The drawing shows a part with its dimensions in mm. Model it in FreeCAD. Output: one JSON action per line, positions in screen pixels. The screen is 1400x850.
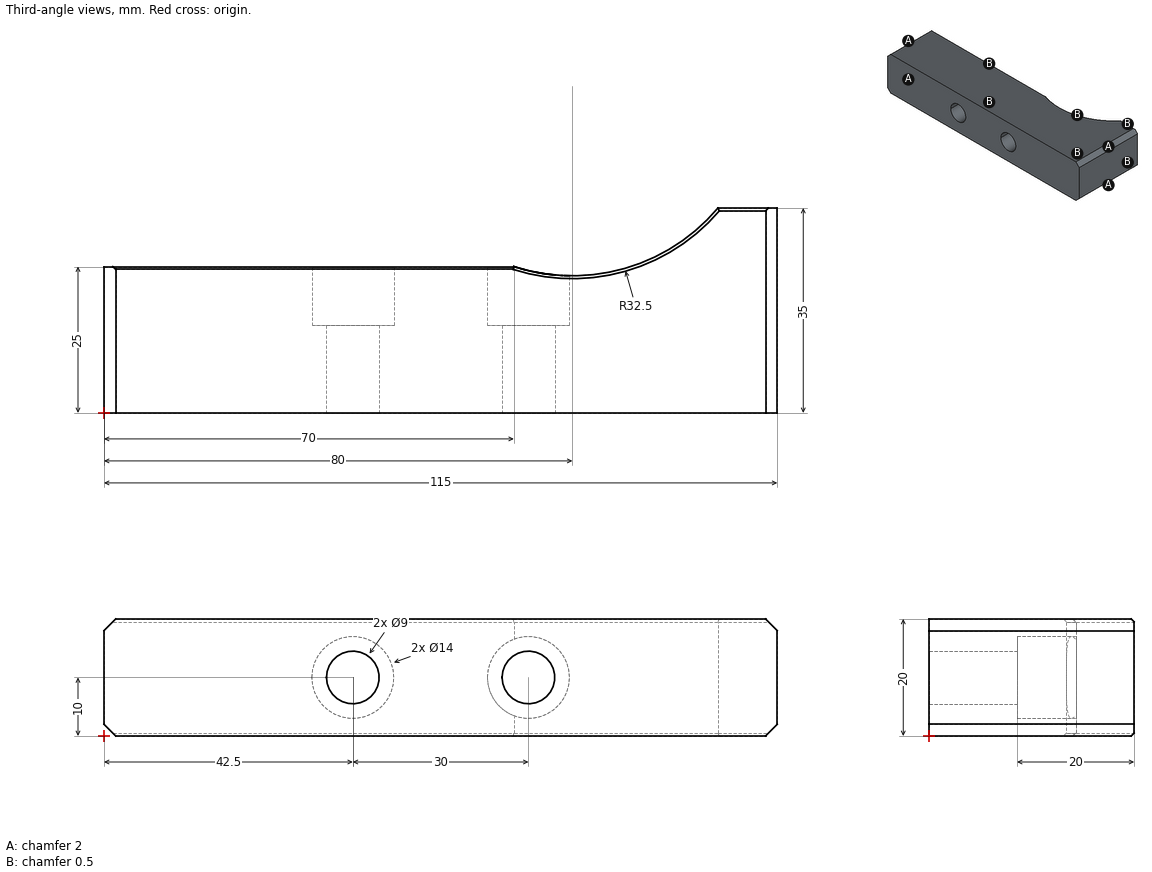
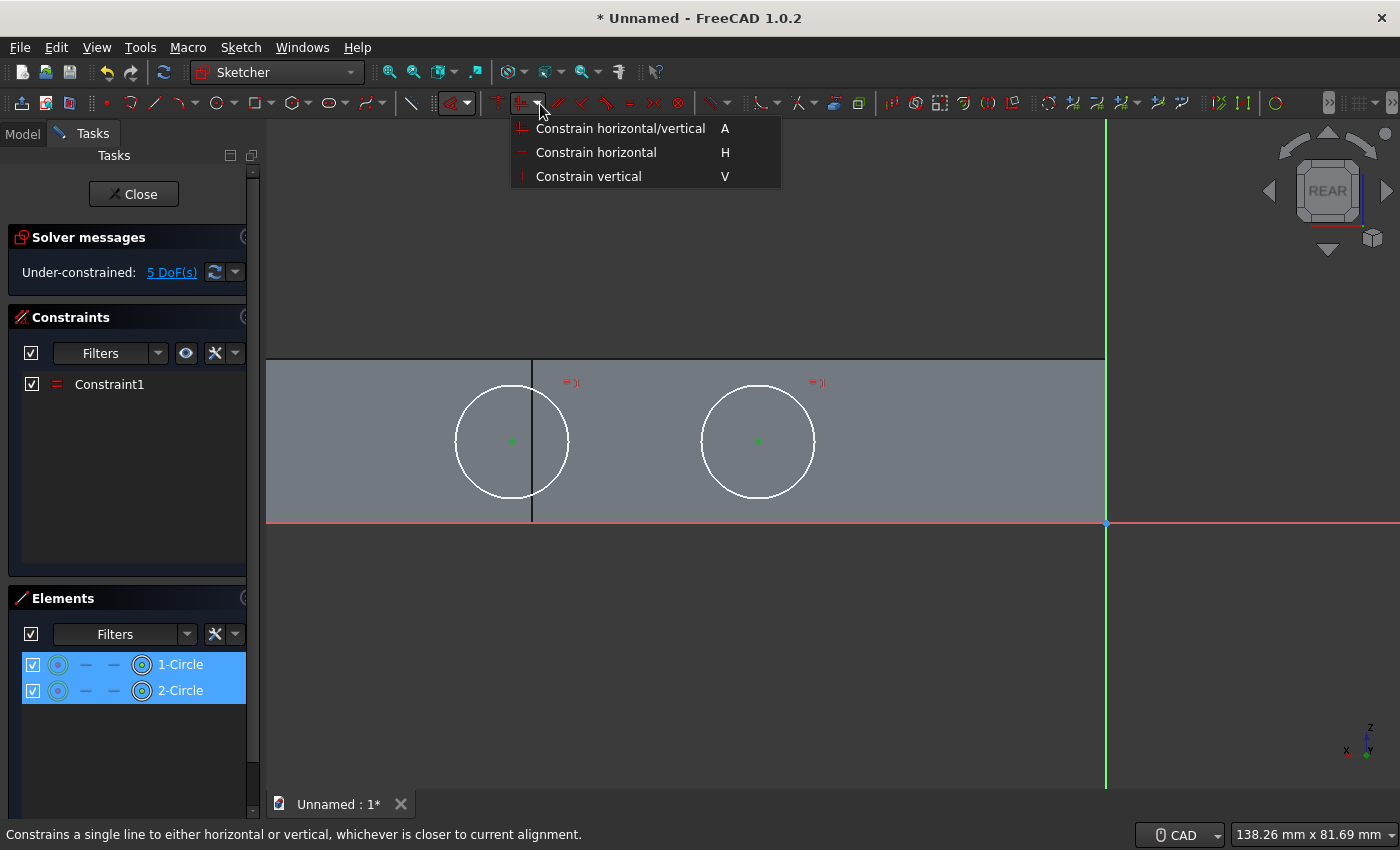
{"action": "left_click", "coordinate": [646, 152]}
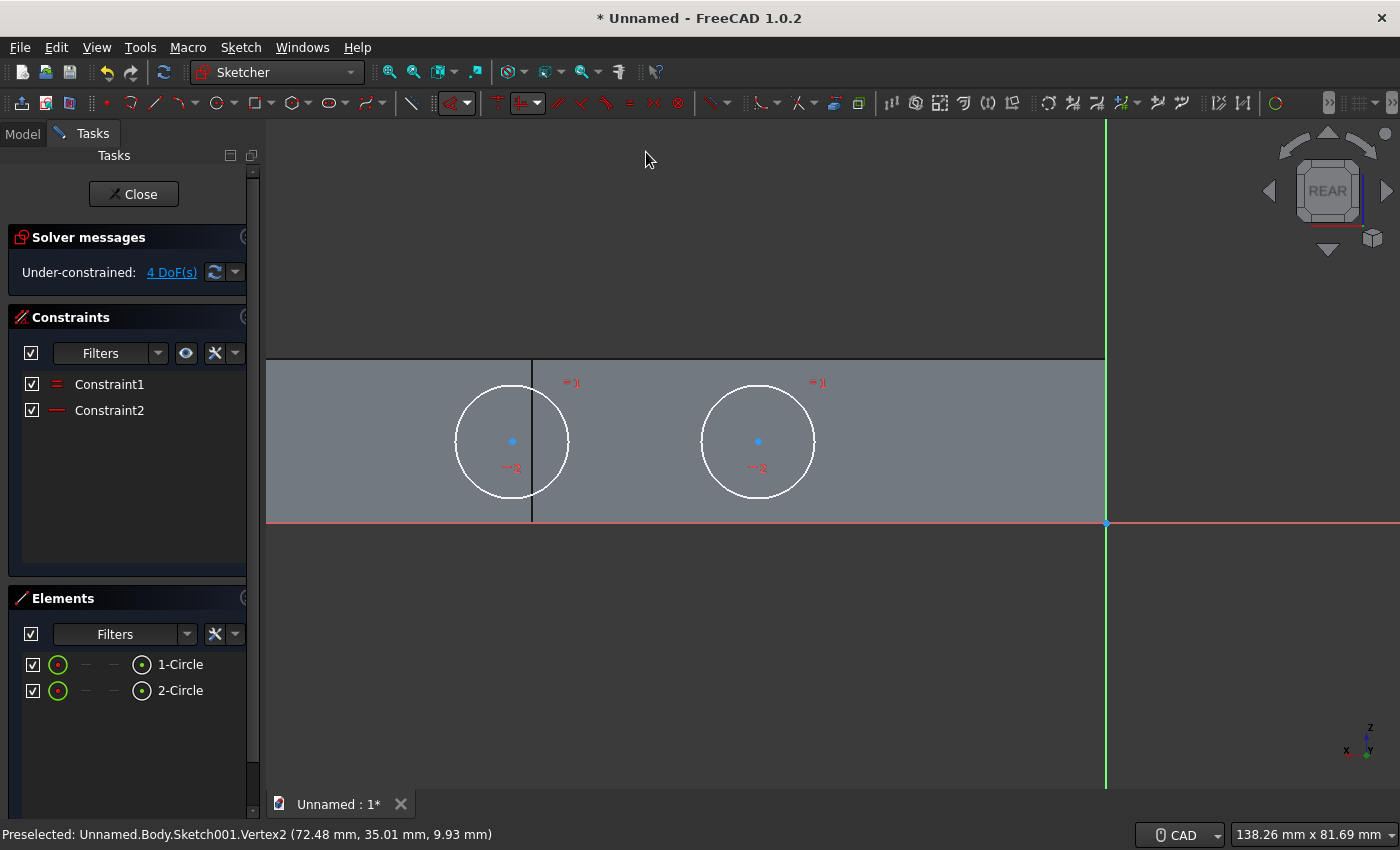
{"action": "left_click", "coordinate": [798, 402]}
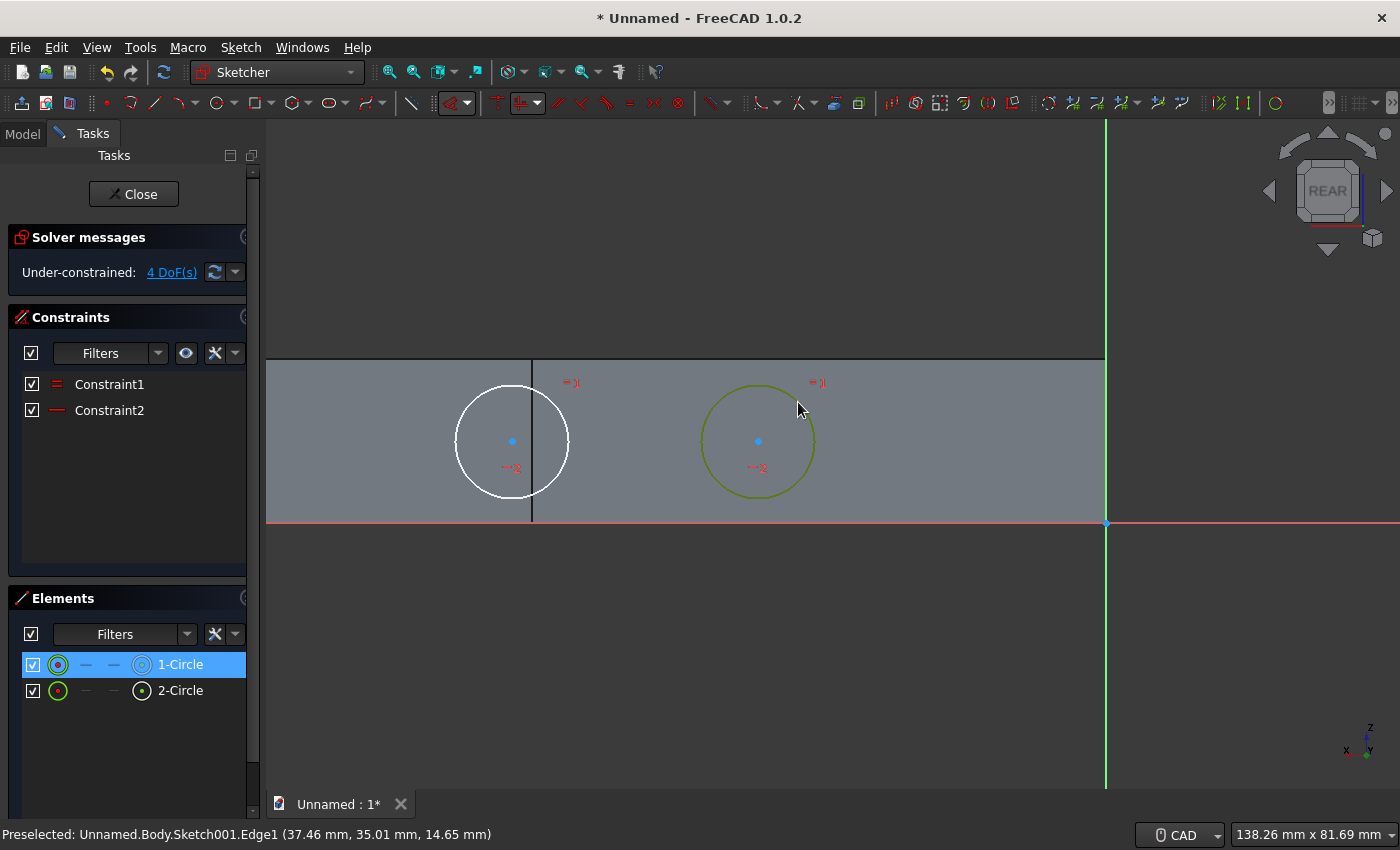
{"action": "left_click", "coordinate": [470, 104]}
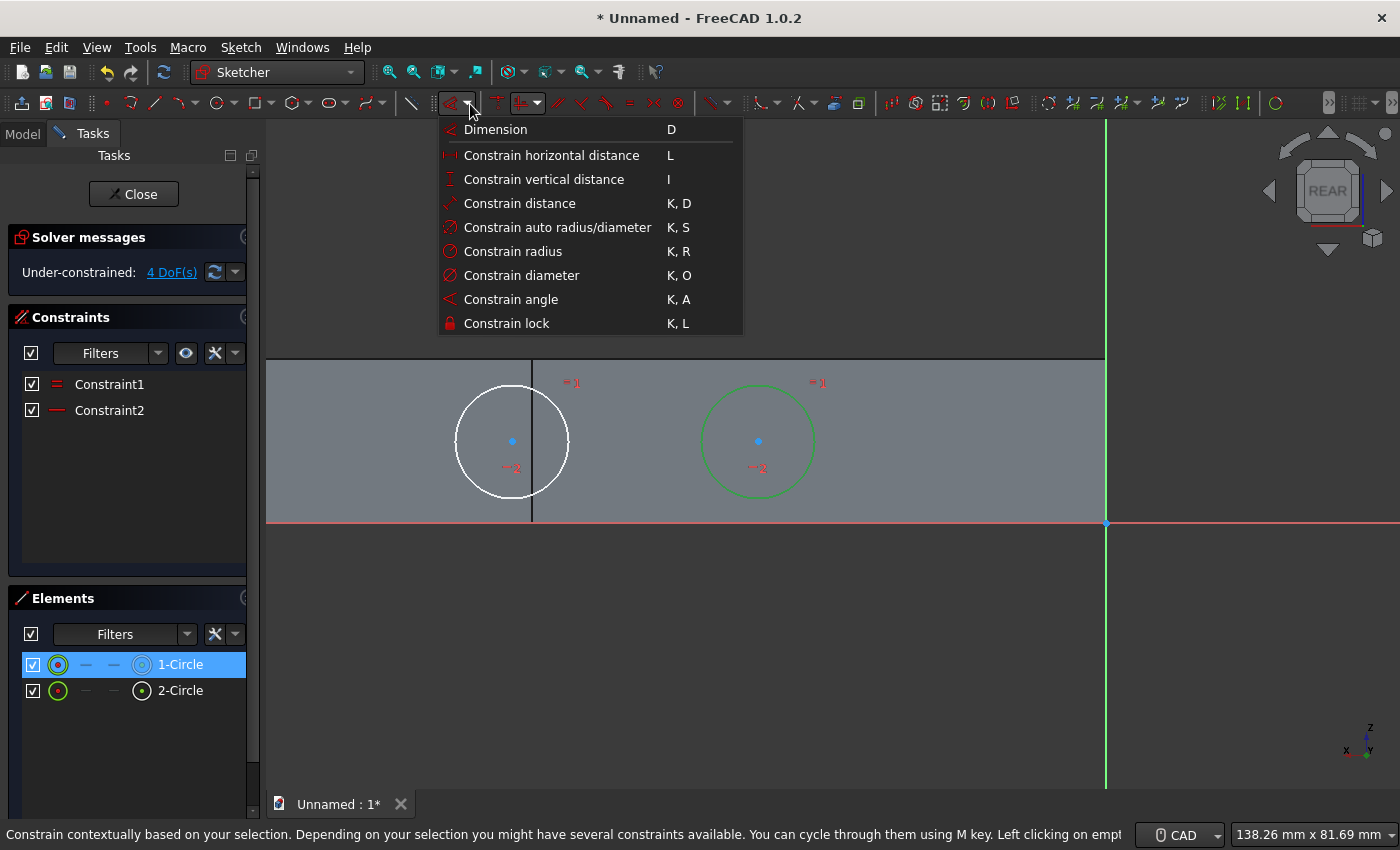
{"action": "left_click", "coordinate": [591, 275]}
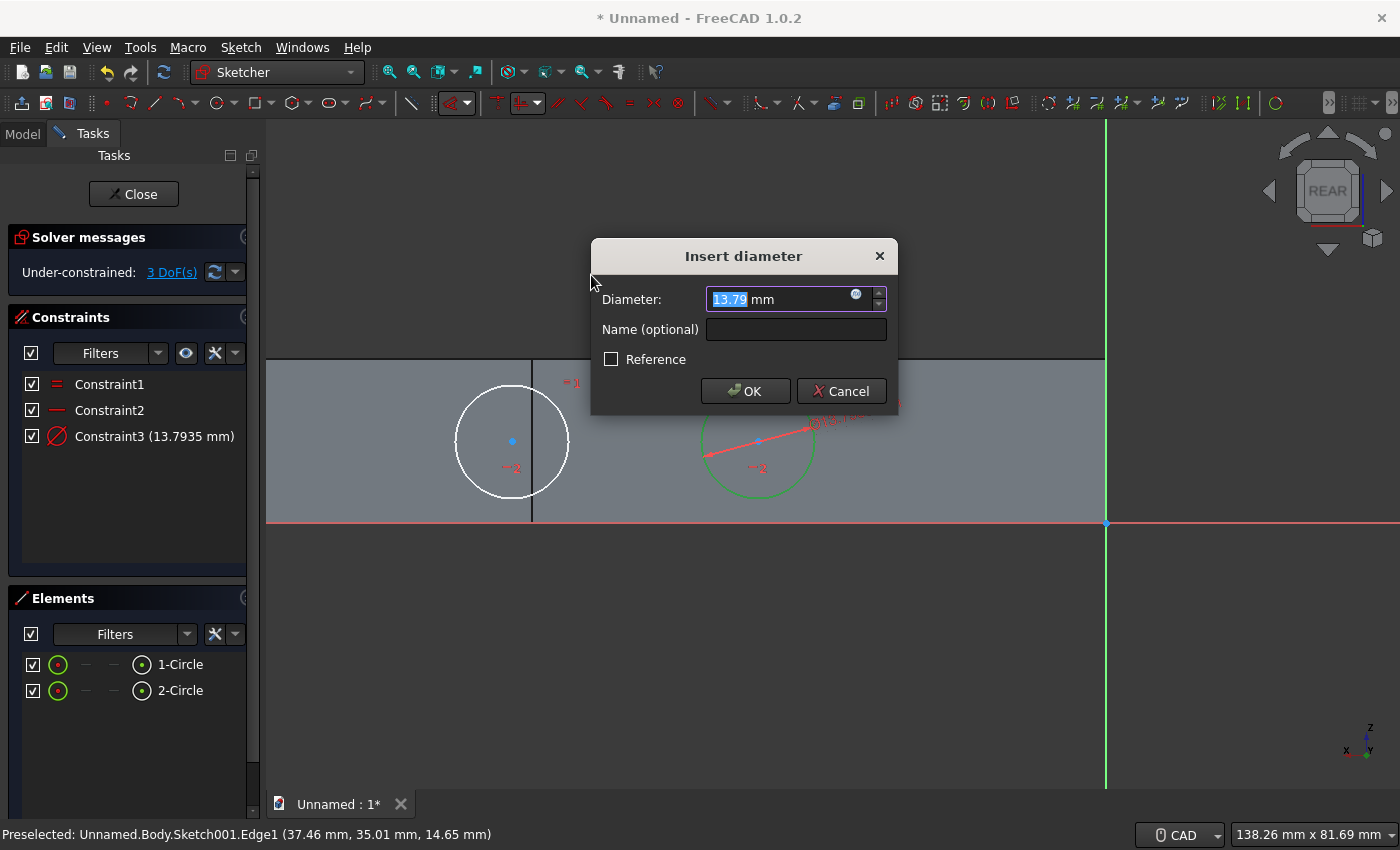
{"action": "type", "text": "14"}
{"action": "key", "text": "Return"}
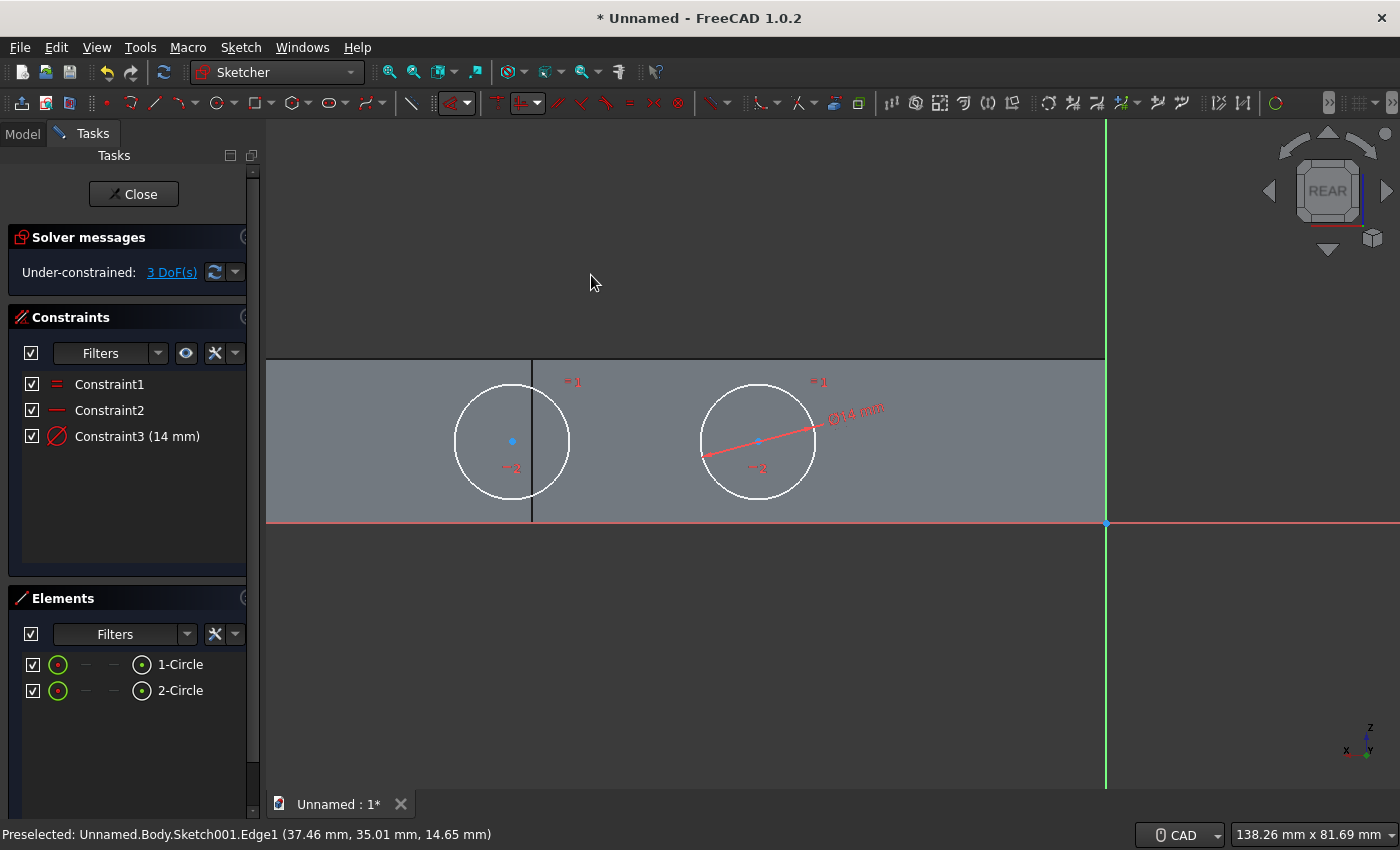
{"action": "left_click", "coordinate": [758, 442]}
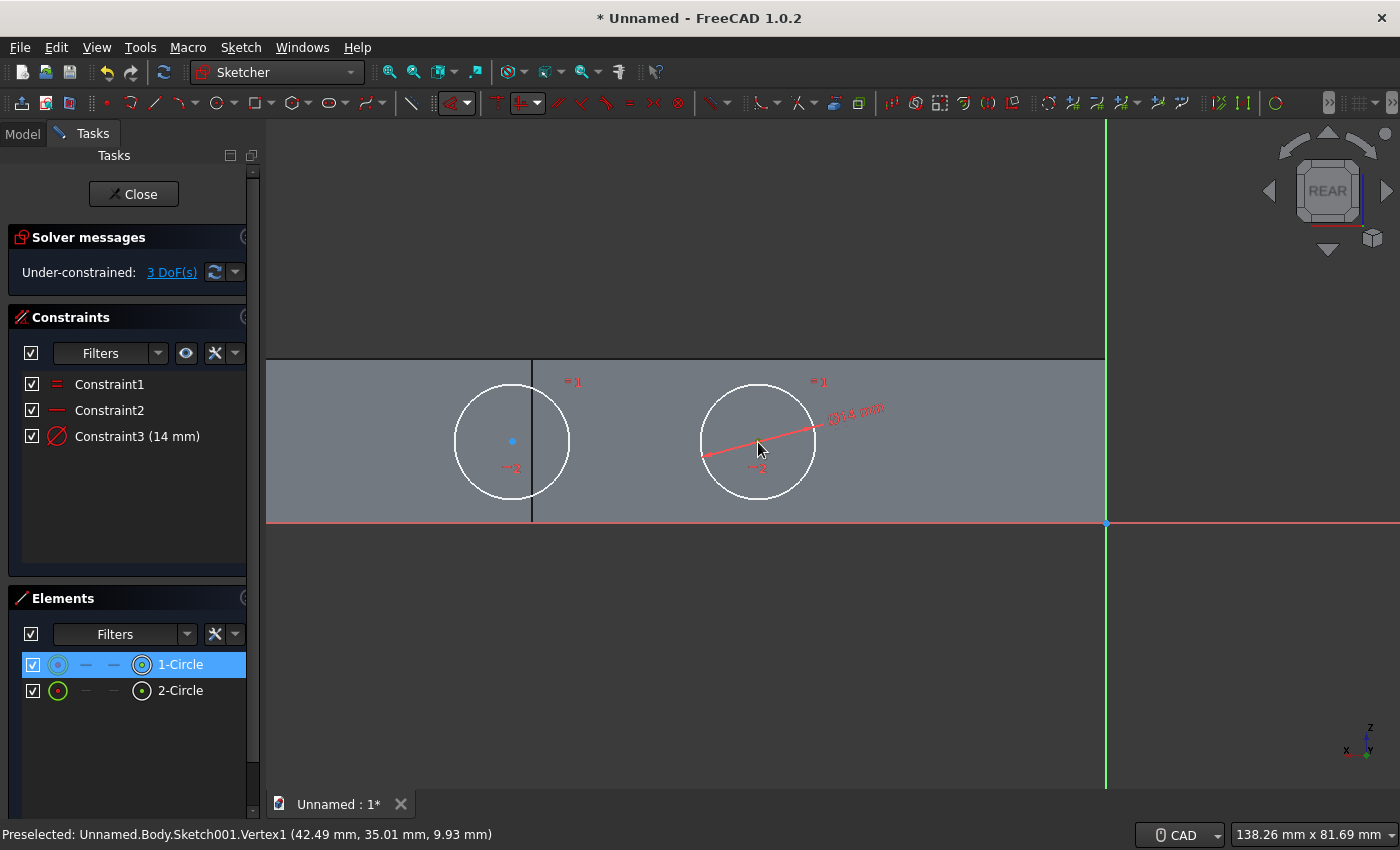
{"action": "key", "text": "i"}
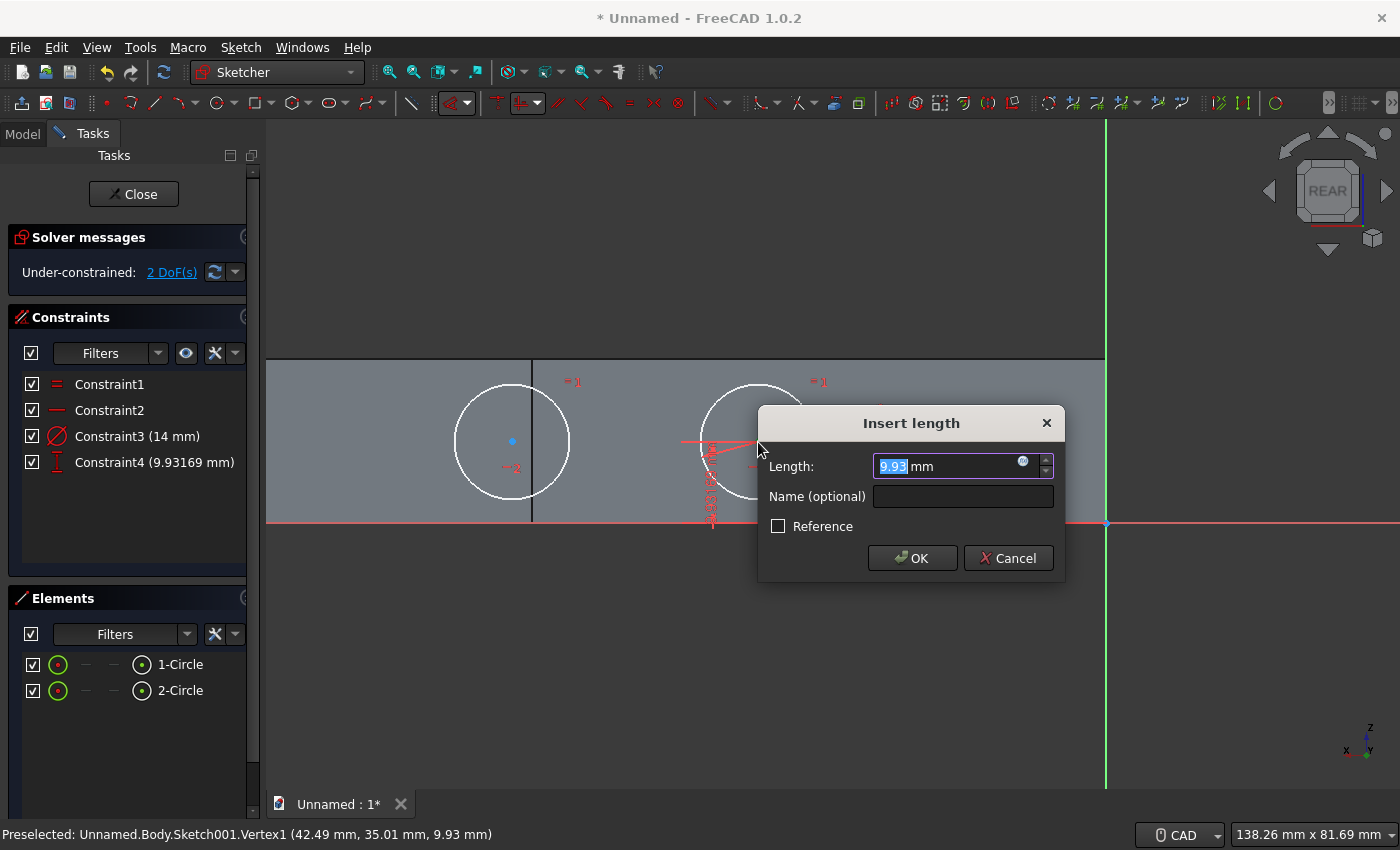
{"action": "type", "text": "10"}
{"action": "key", "text": "Return"}